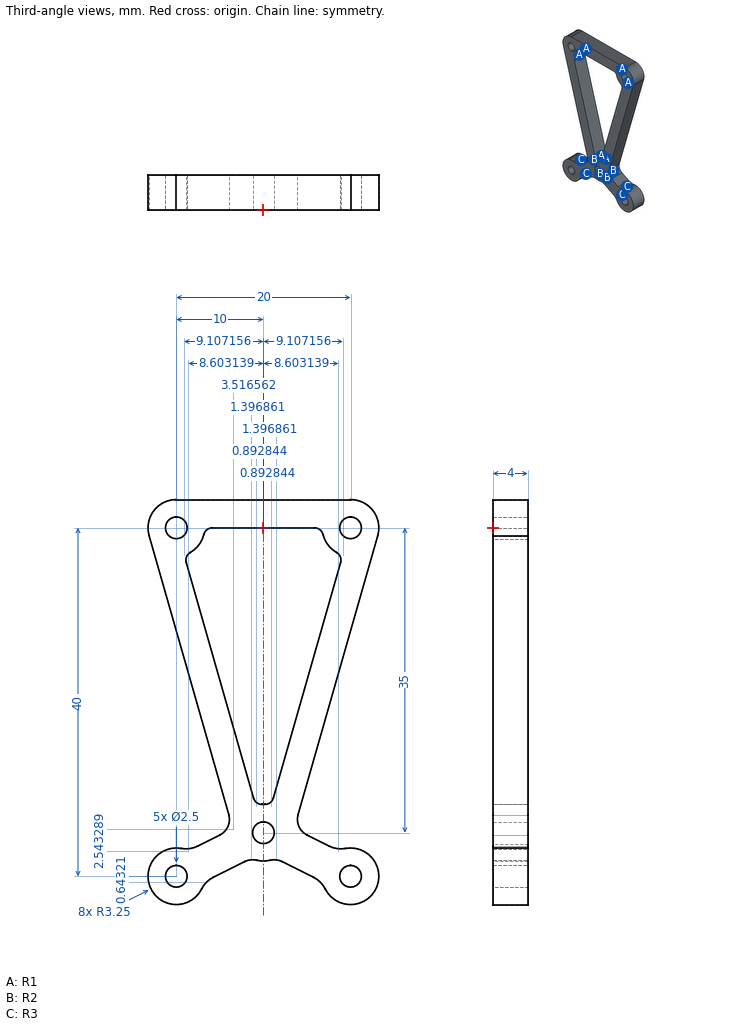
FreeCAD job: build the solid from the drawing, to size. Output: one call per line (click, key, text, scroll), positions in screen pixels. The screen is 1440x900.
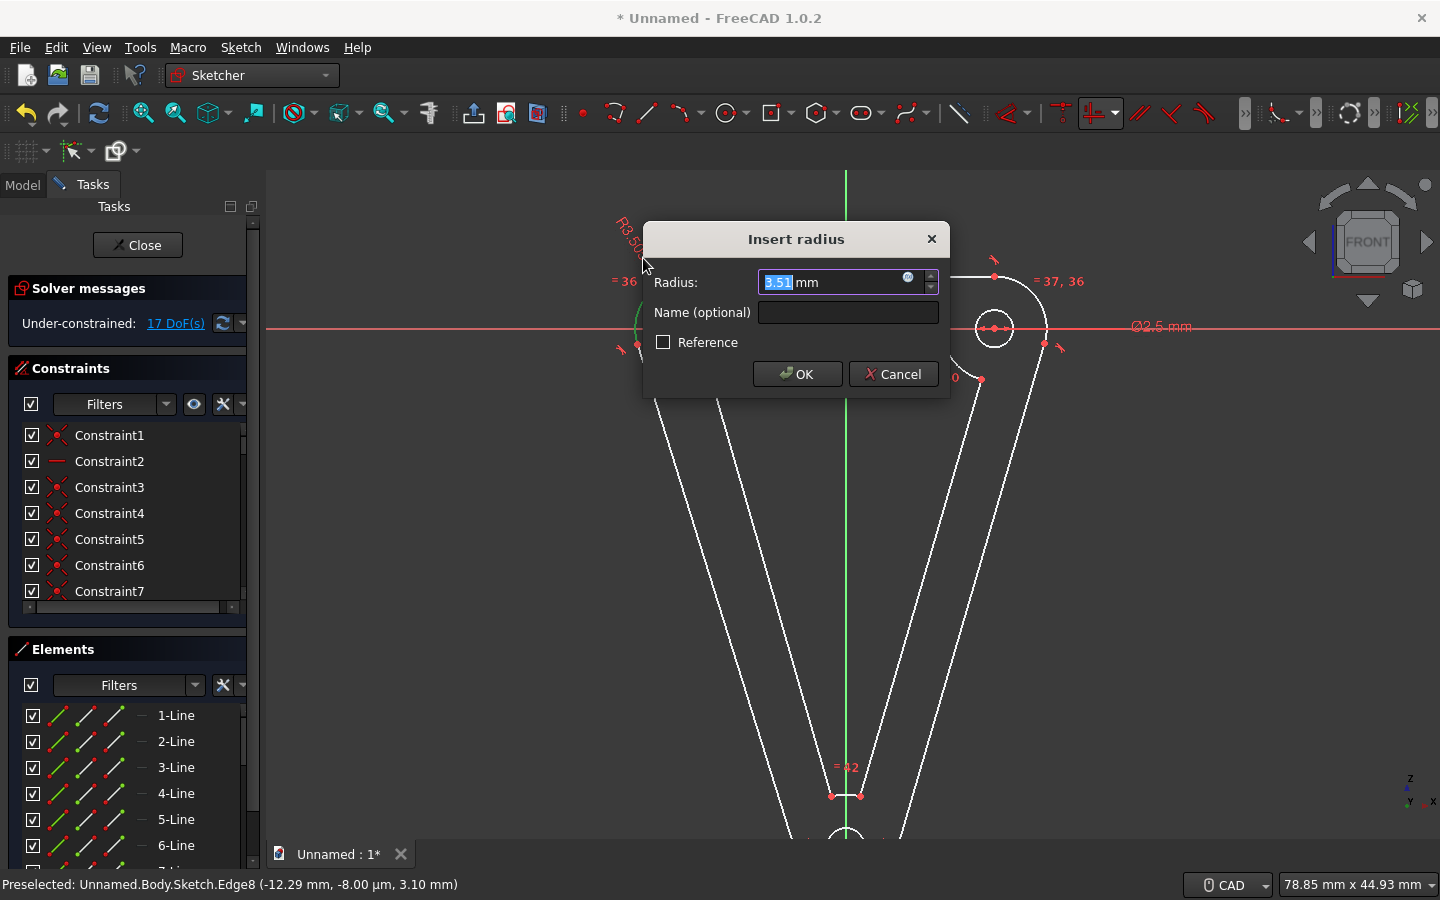
text(3.25)
key(Return)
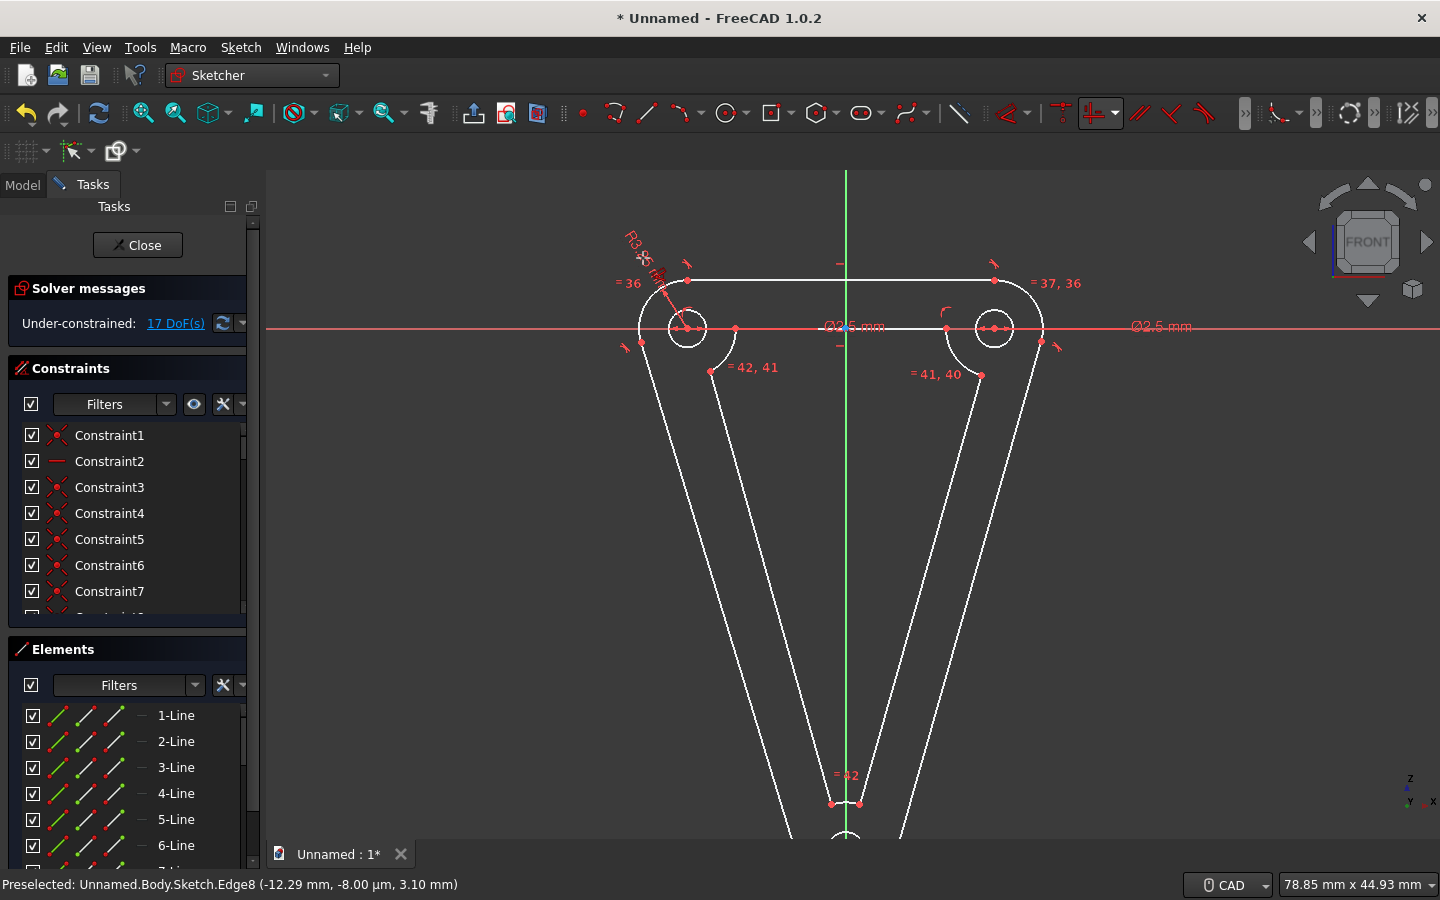
click(780, 280)
click(770, 246)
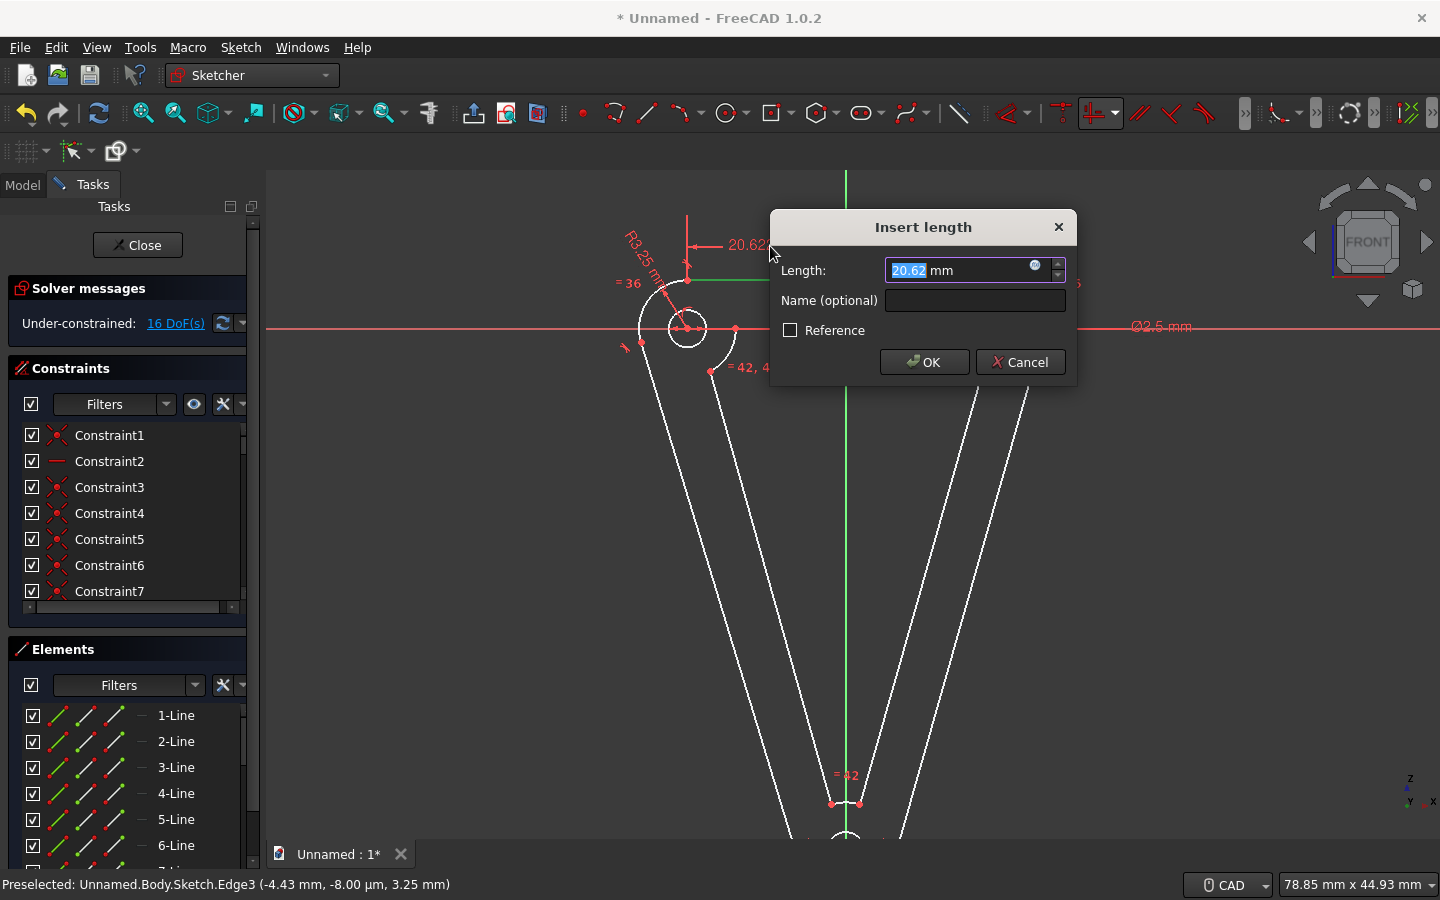
text(20)
key(Return)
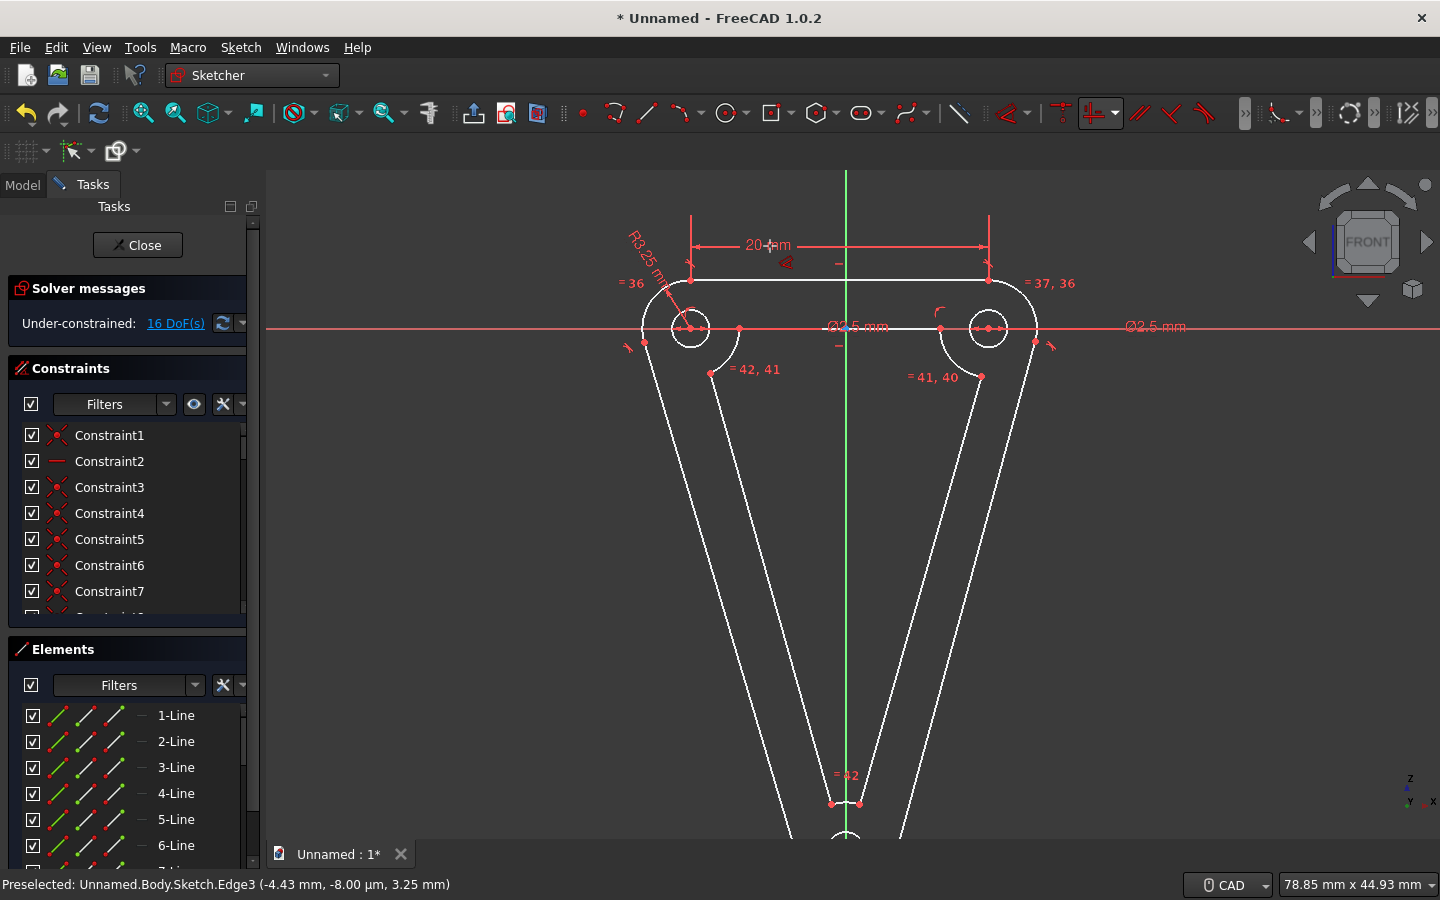
scroll(660, 284, down, 2)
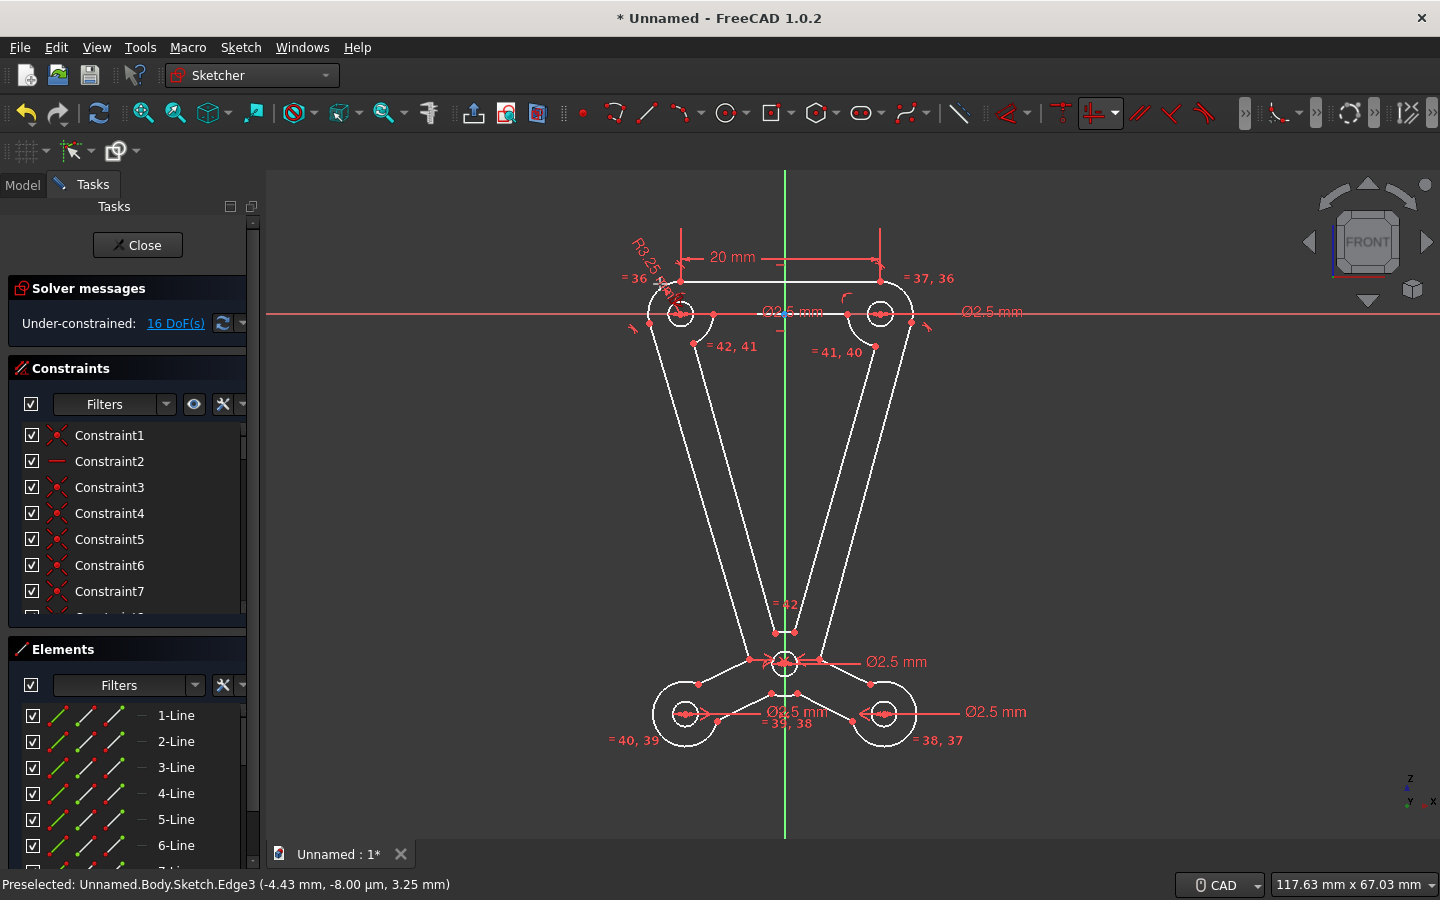
click(685, 714)
click(735, 748)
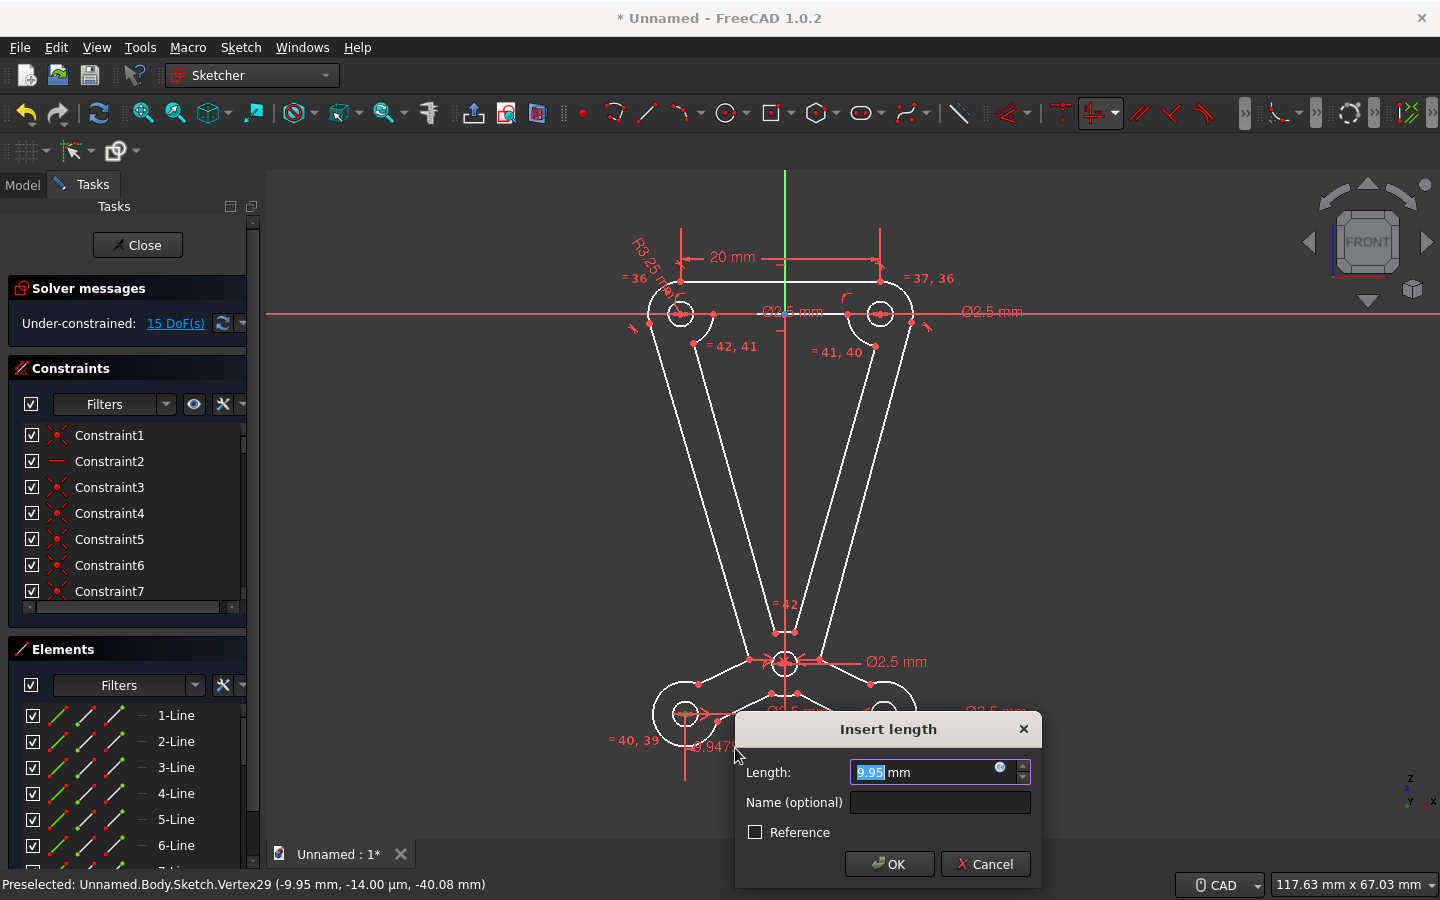
text(10)
key(Return)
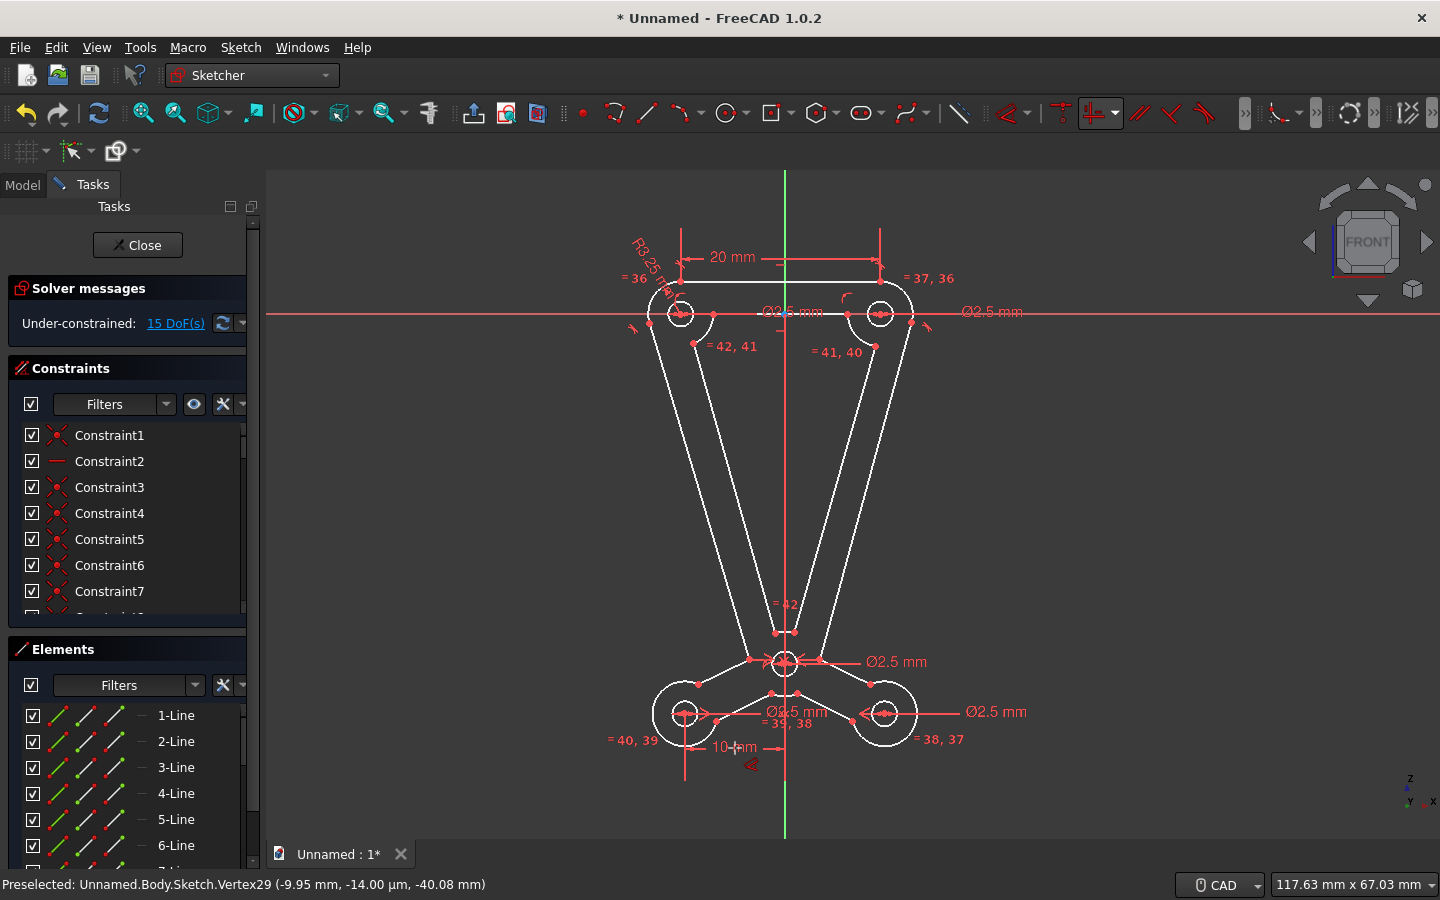
click(685, 714)
click(651, 514)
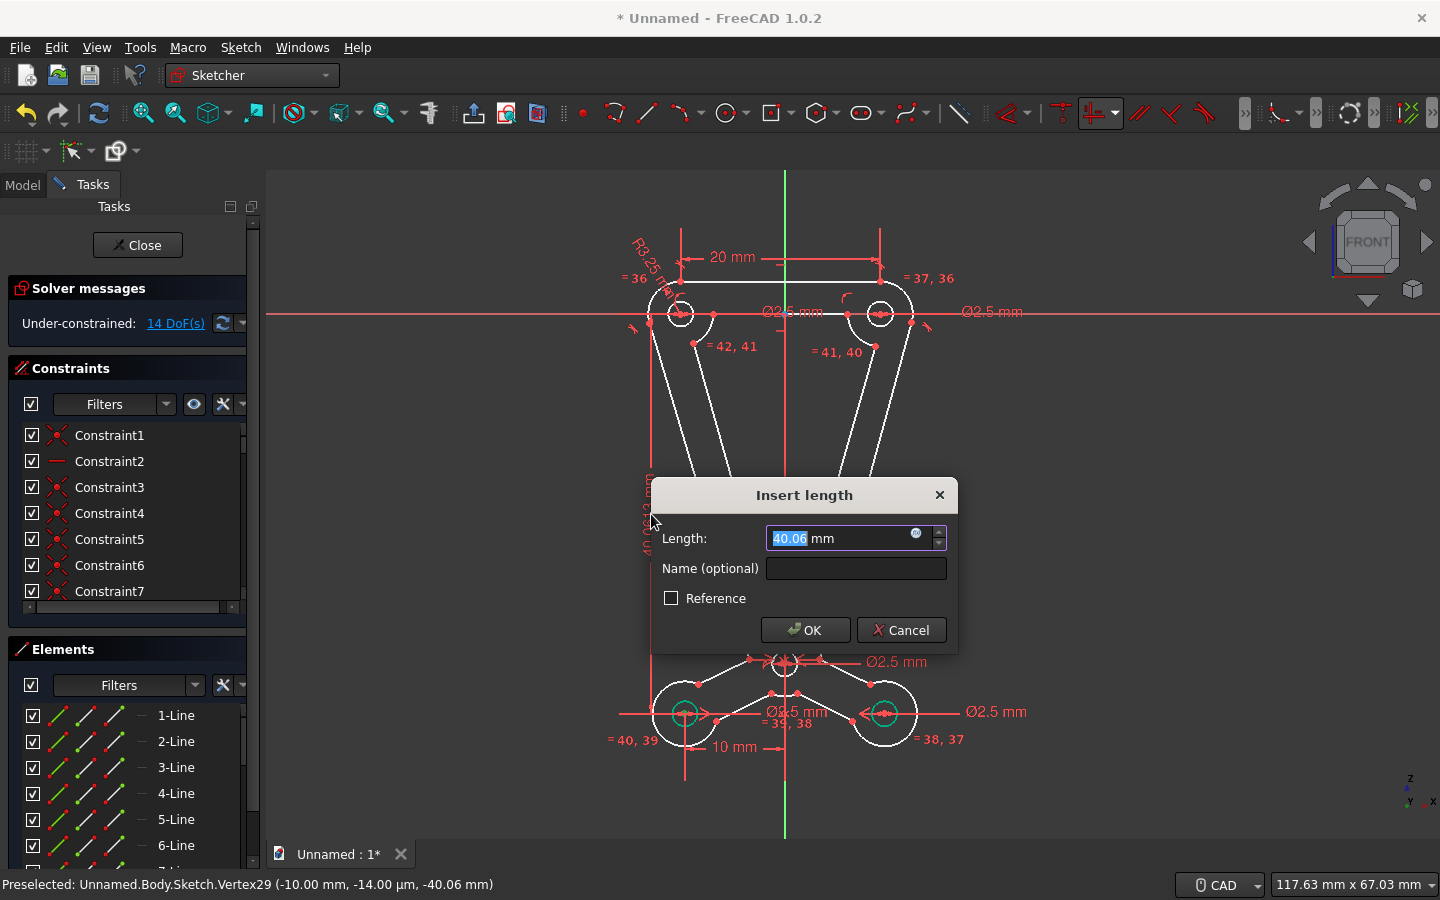
text(40)
key(Return)